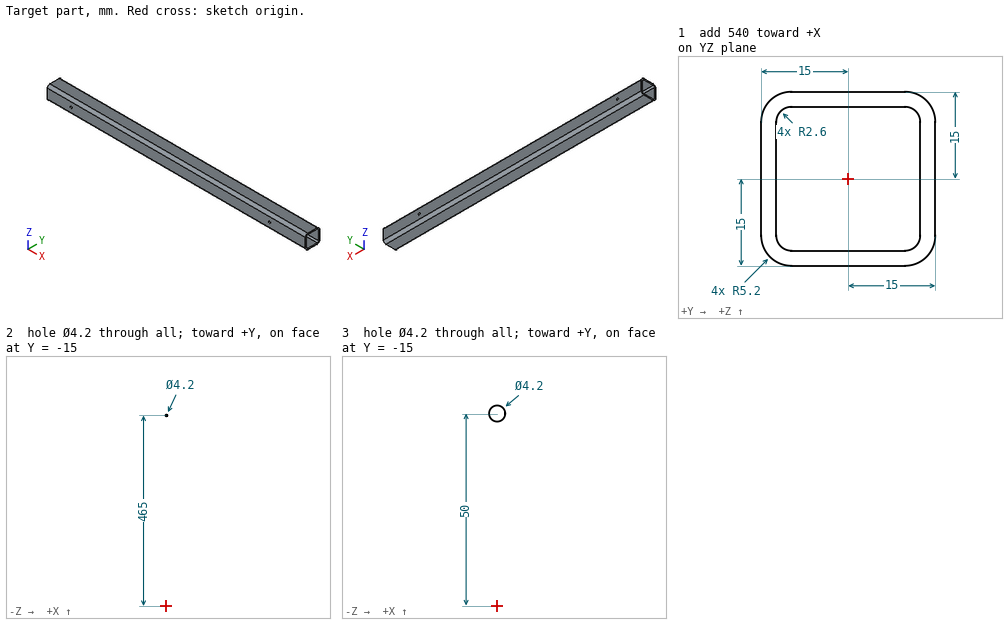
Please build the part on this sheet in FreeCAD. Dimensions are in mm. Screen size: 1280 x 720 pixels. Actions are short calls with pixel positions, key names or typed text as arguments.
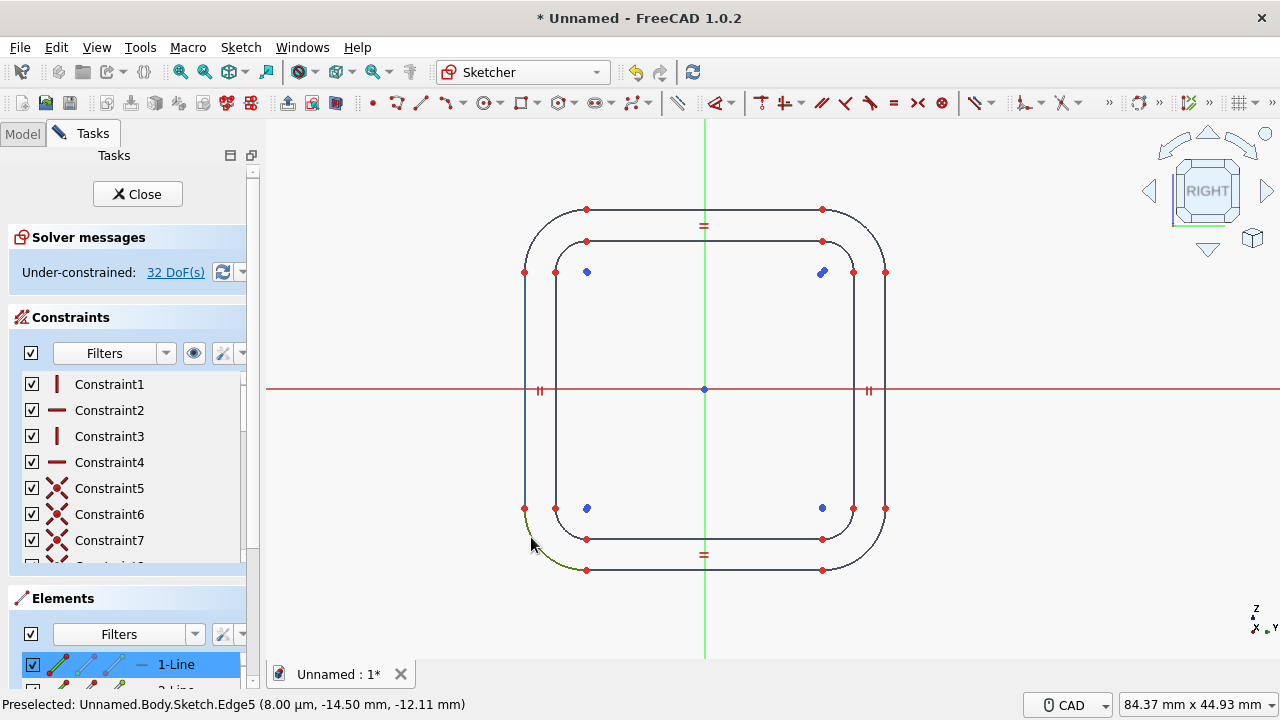
click(870, 104)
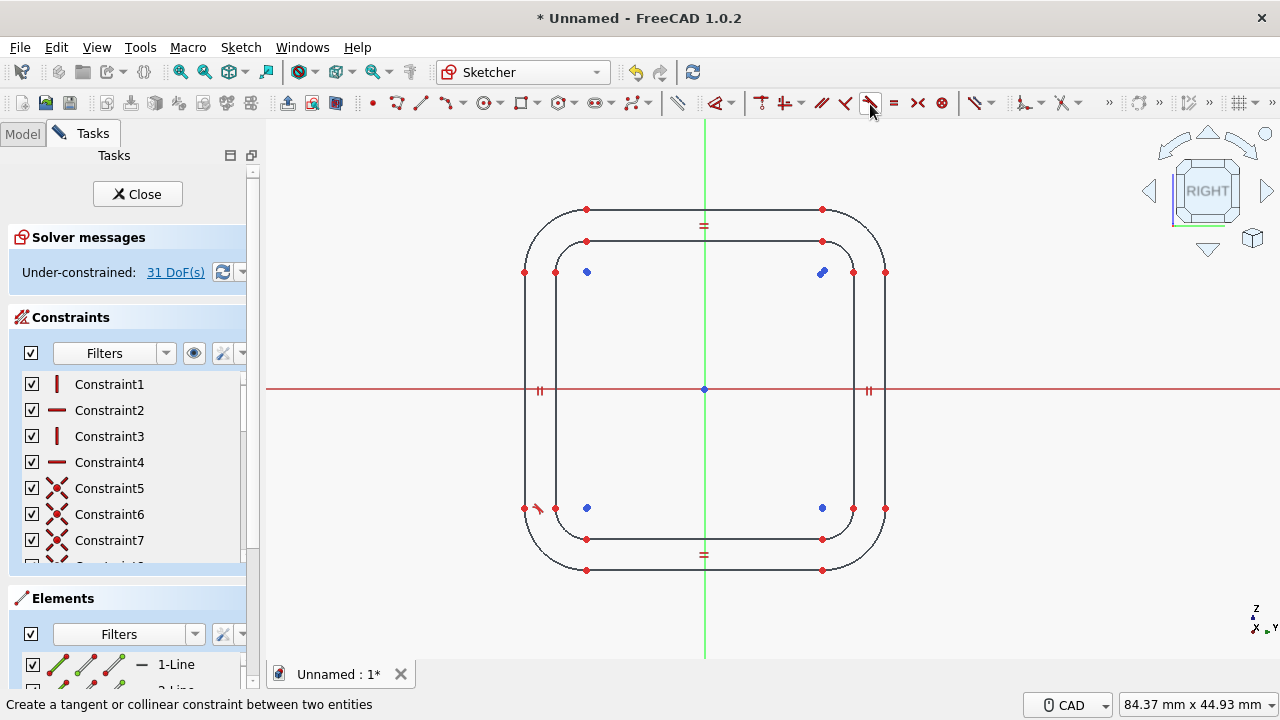
click(525, 343)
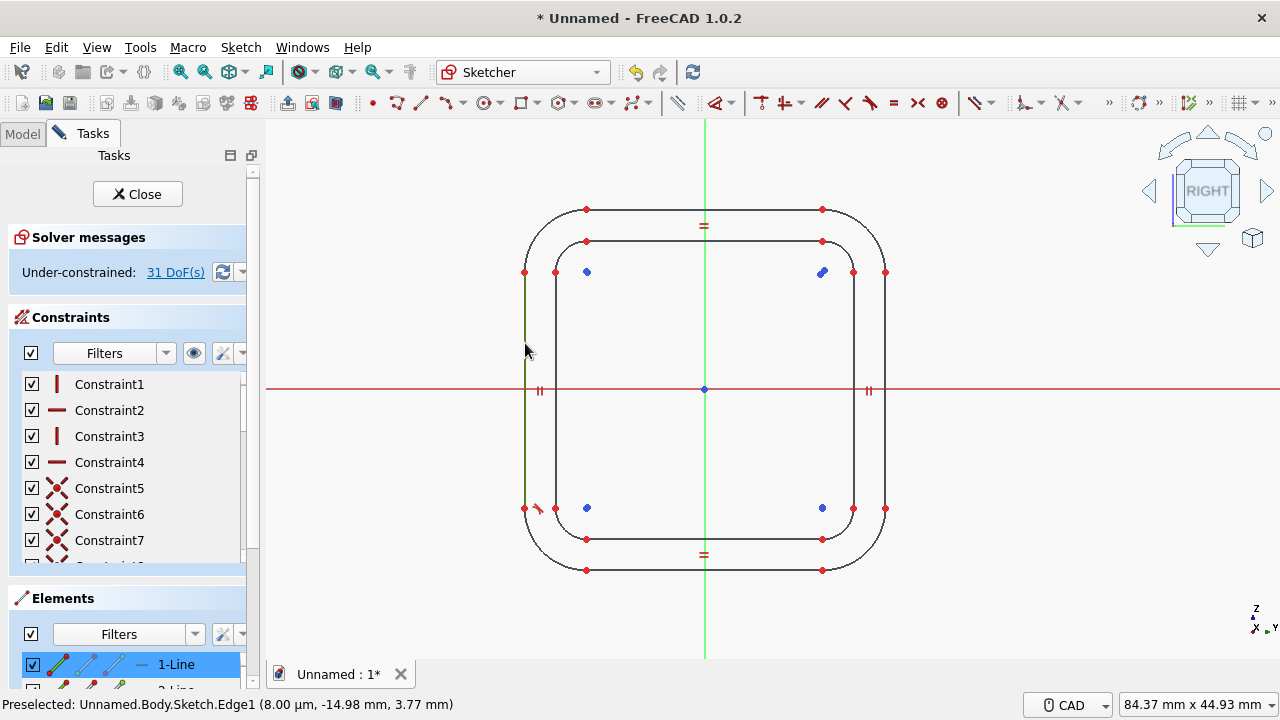
click(559, 217)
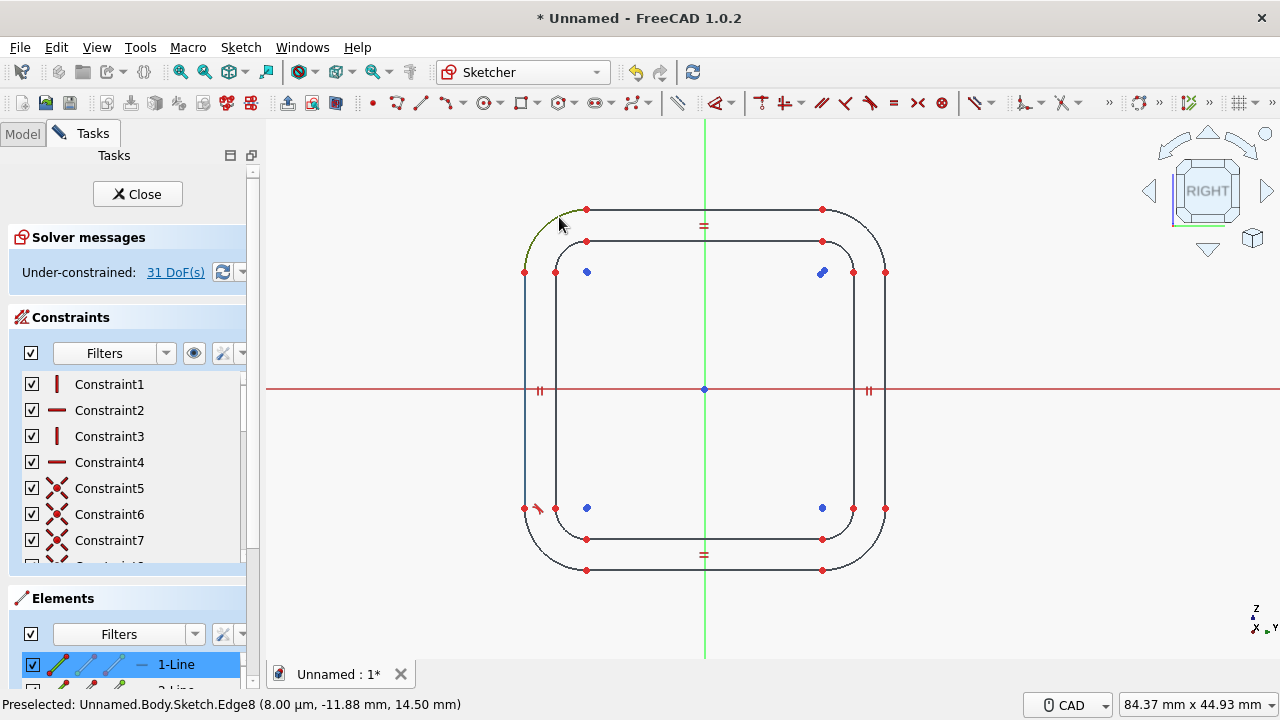
key(t)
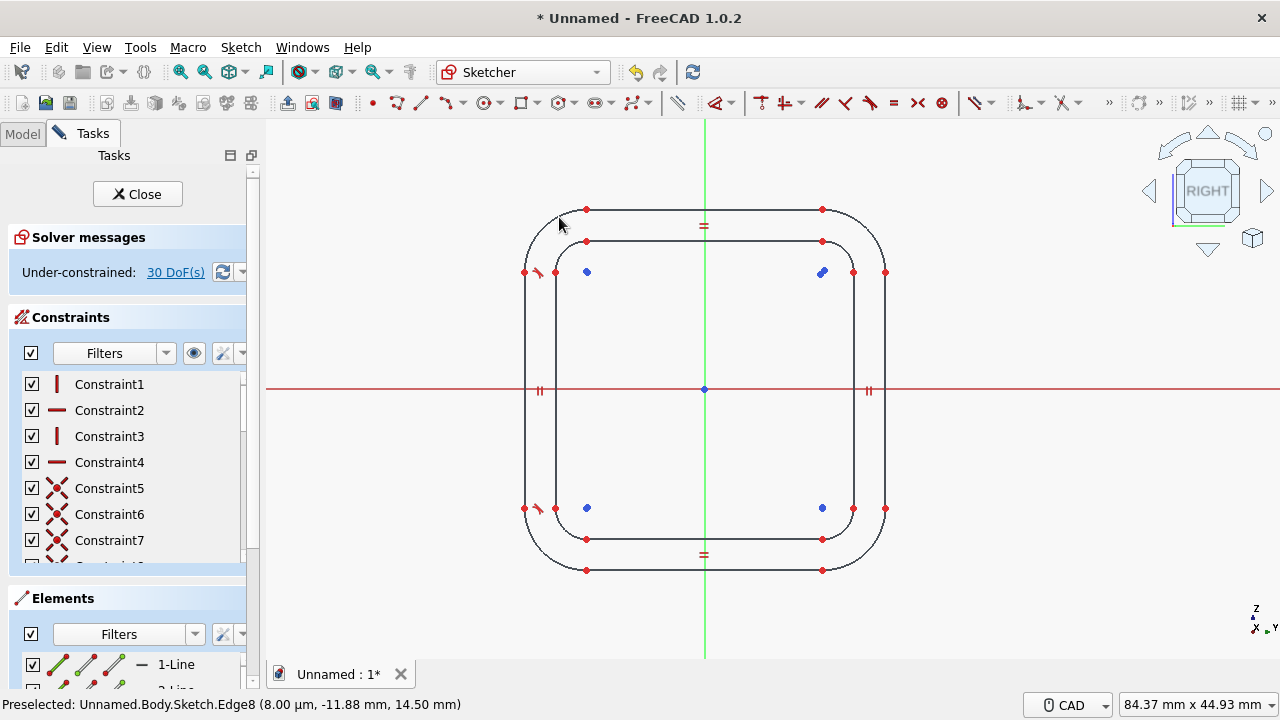
click(657, 570)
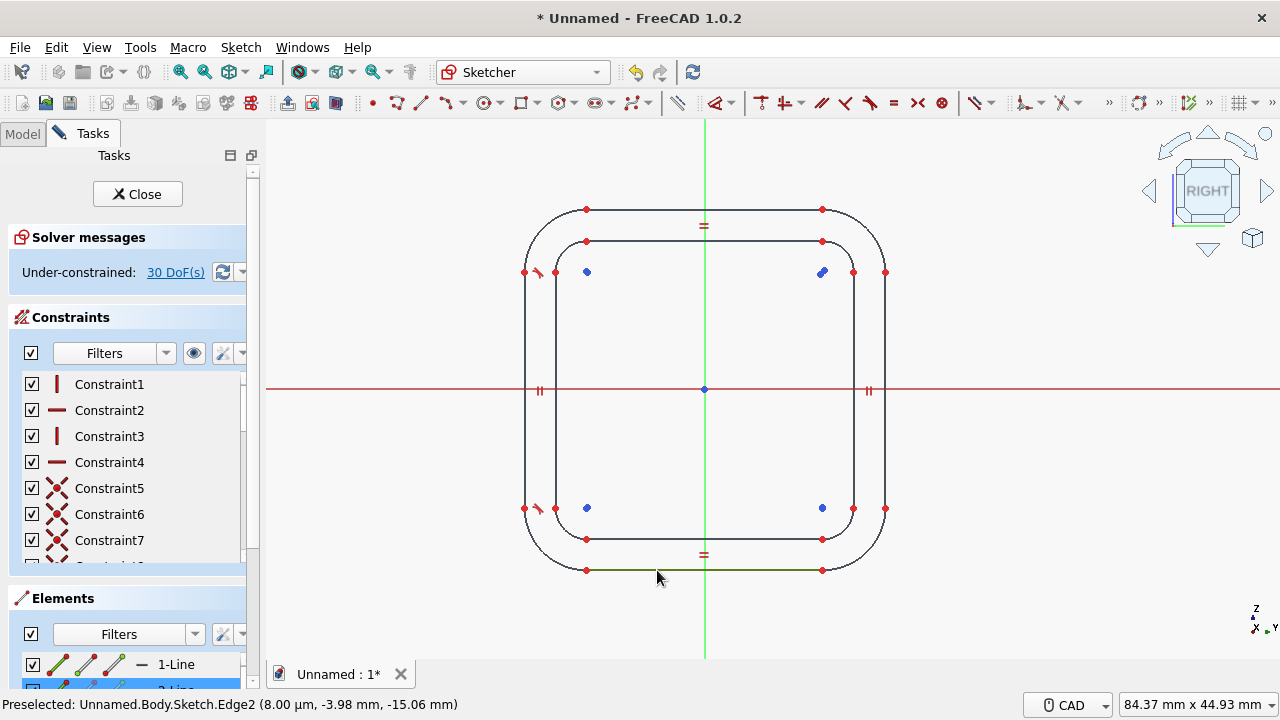
click(532, 537)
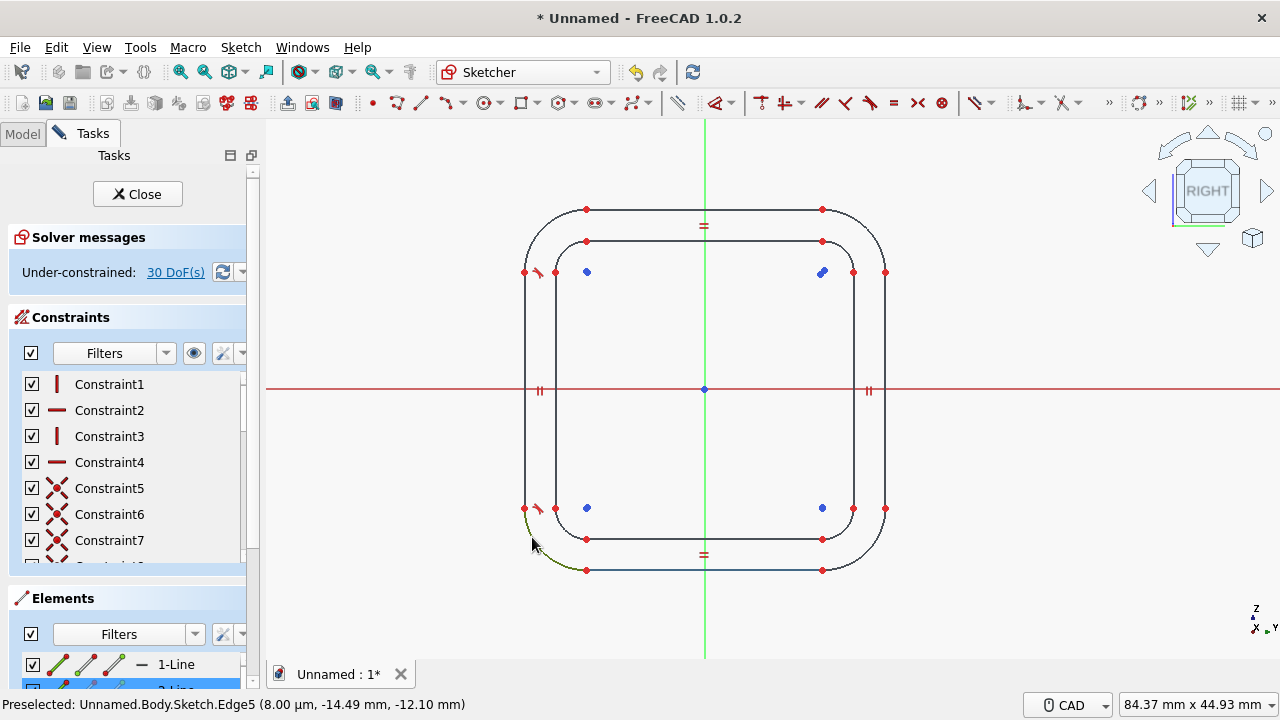
click(870, 104)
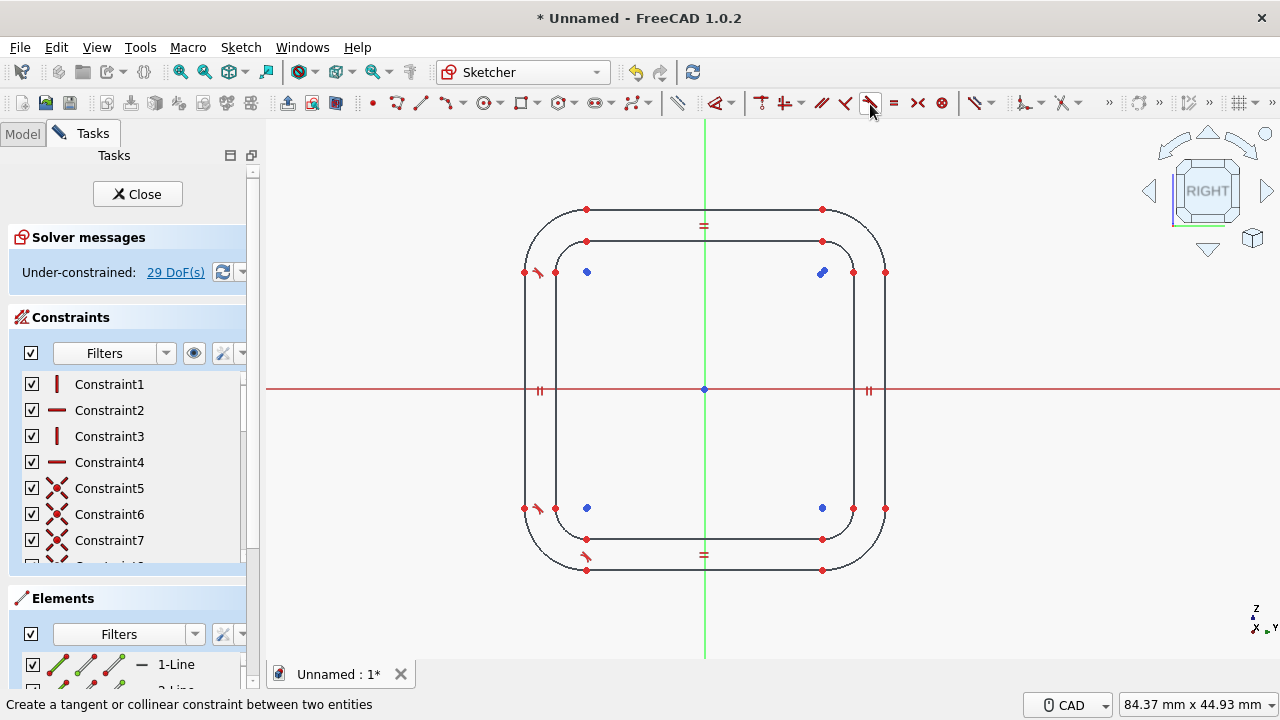
click(657, 570)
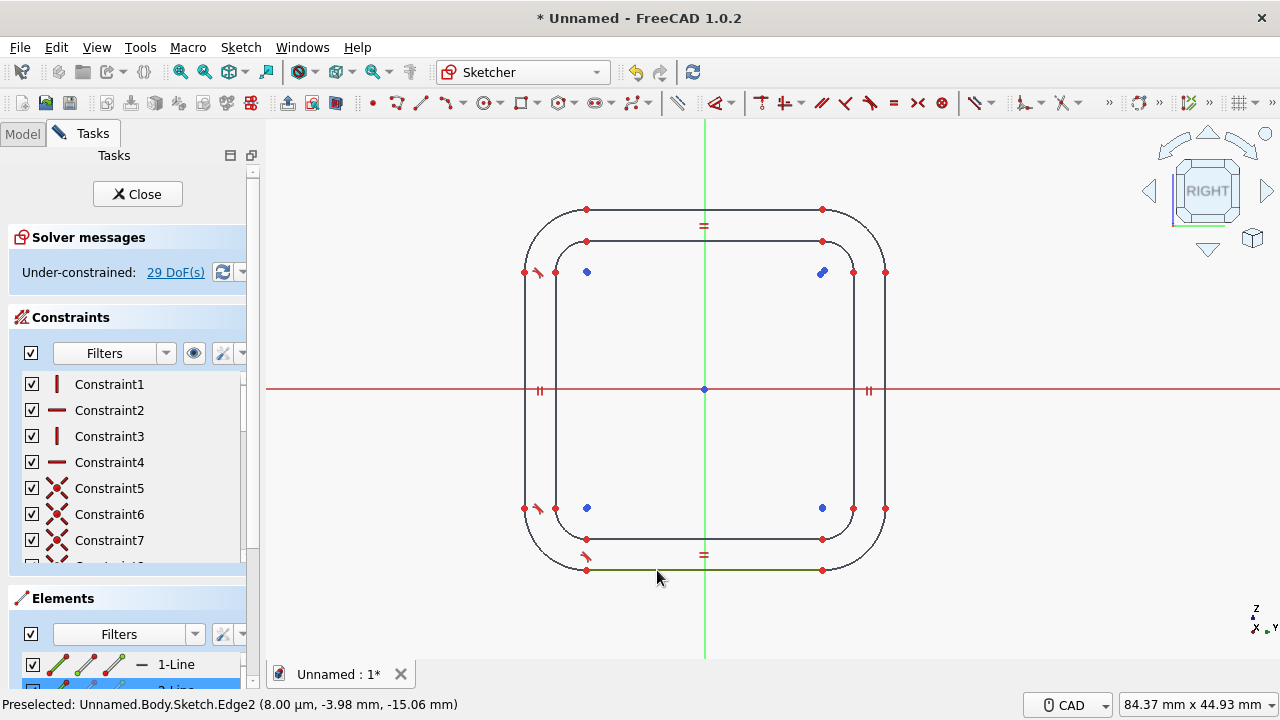
click(851, 563)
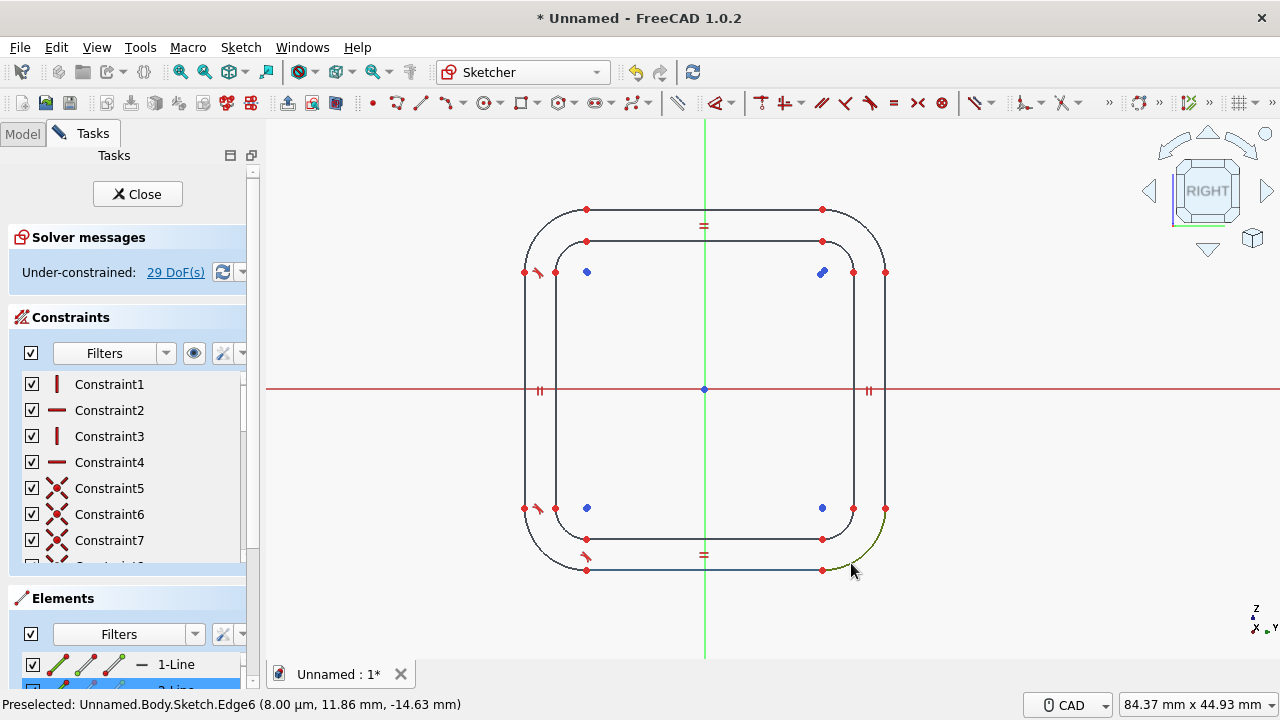
click(870, 104)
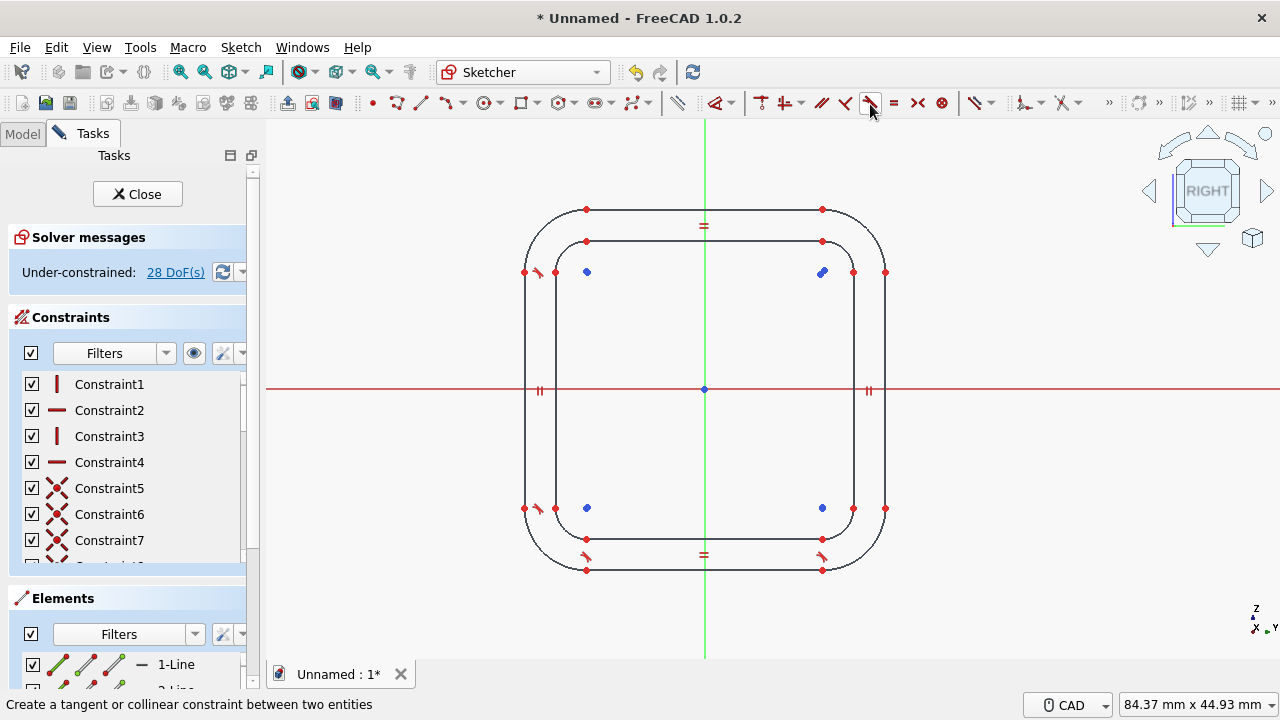
click(885, 438)